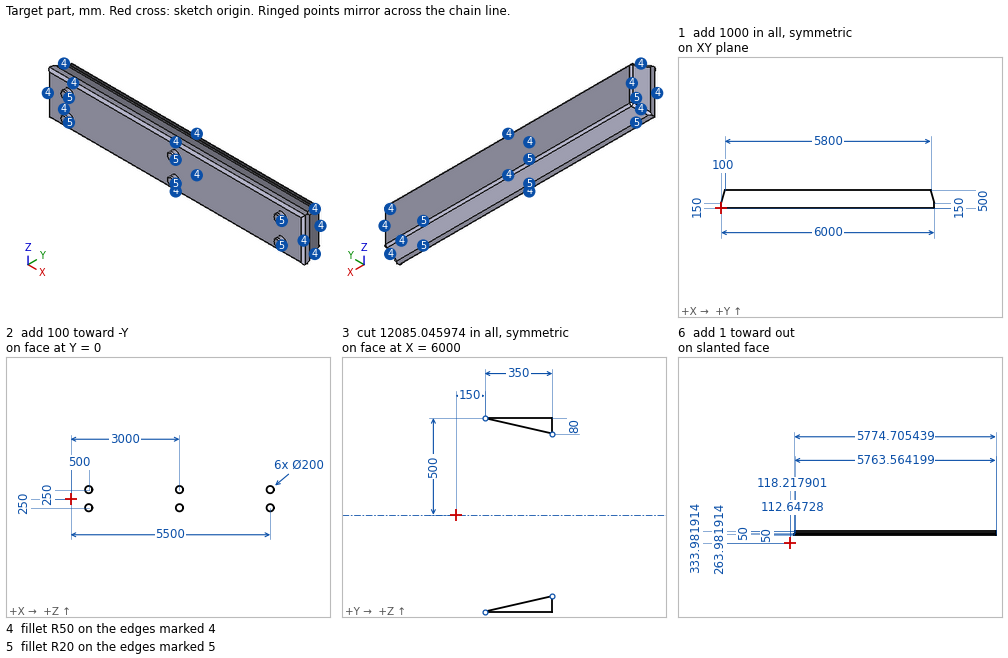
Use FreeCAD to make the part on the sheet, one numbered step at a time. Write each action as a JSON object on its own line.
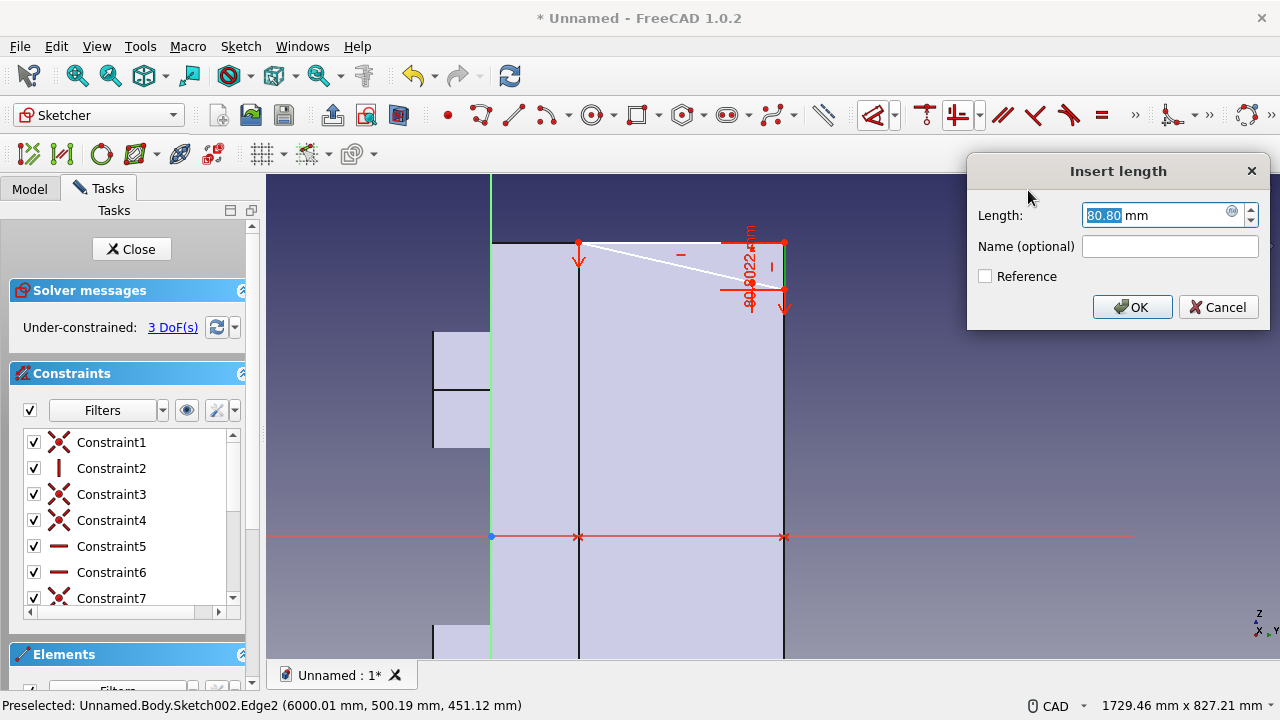
{"action": "type", "text": "80"}
{"action": "key", "text": "Return"}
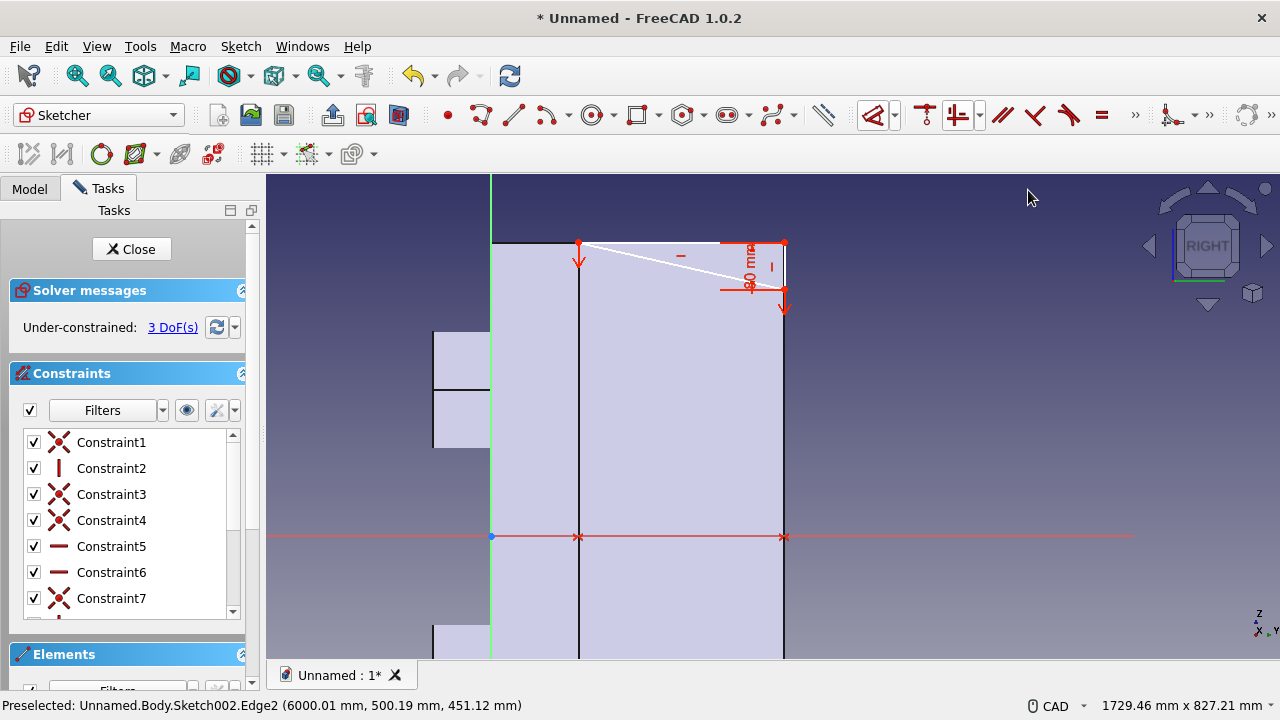
{"action": "left_click", "coordinate": [723, 243]}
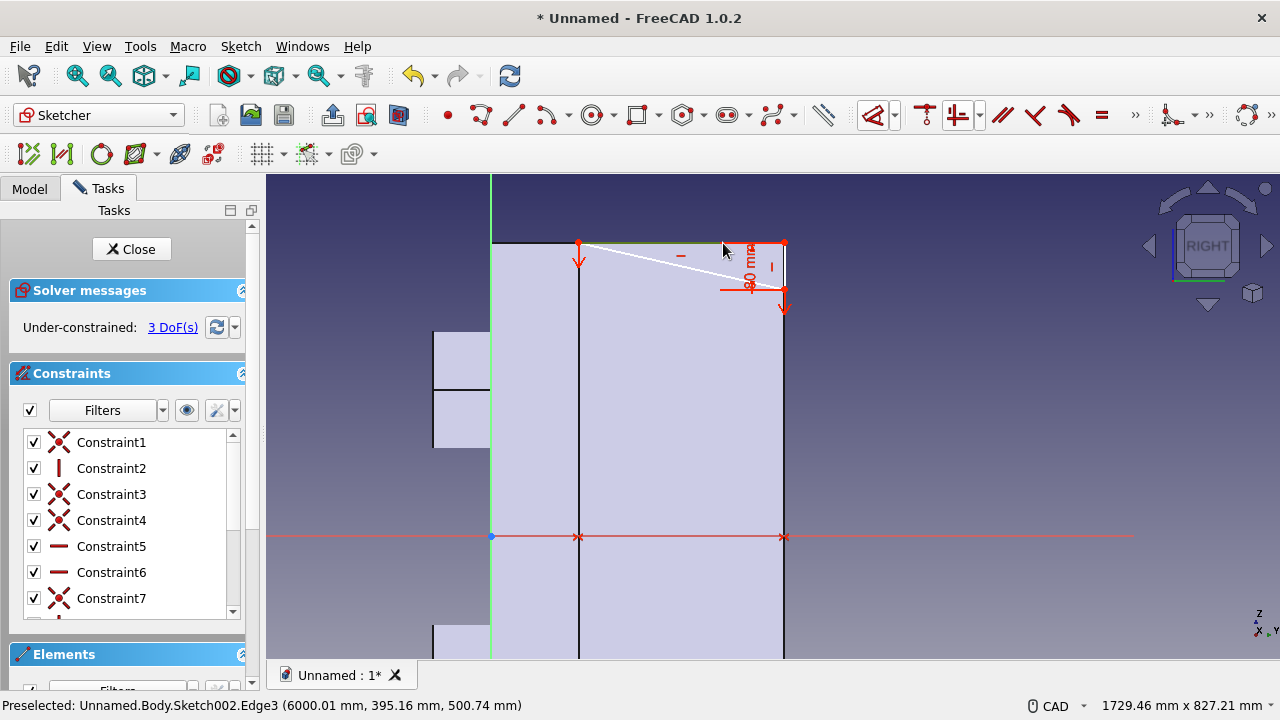
{"action": "key", "text": "l"}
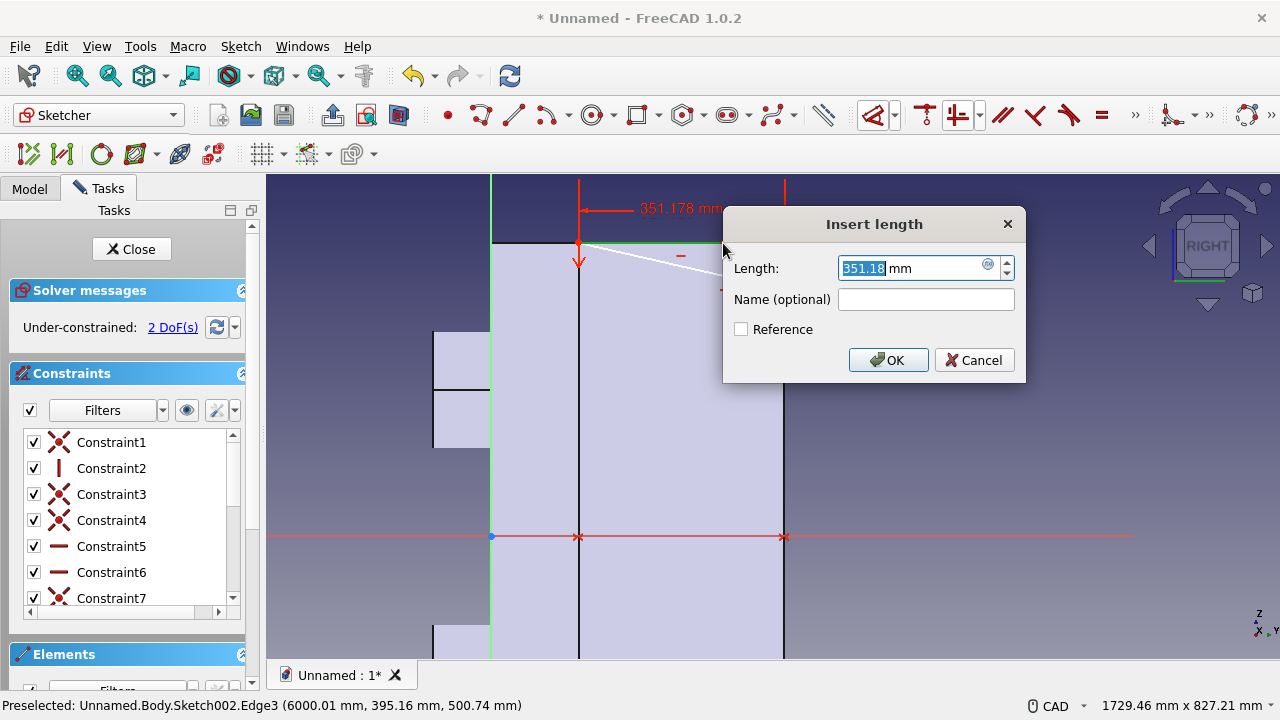
{"action": "type", "text": "350"}
{"action": "key", "text": "Return"}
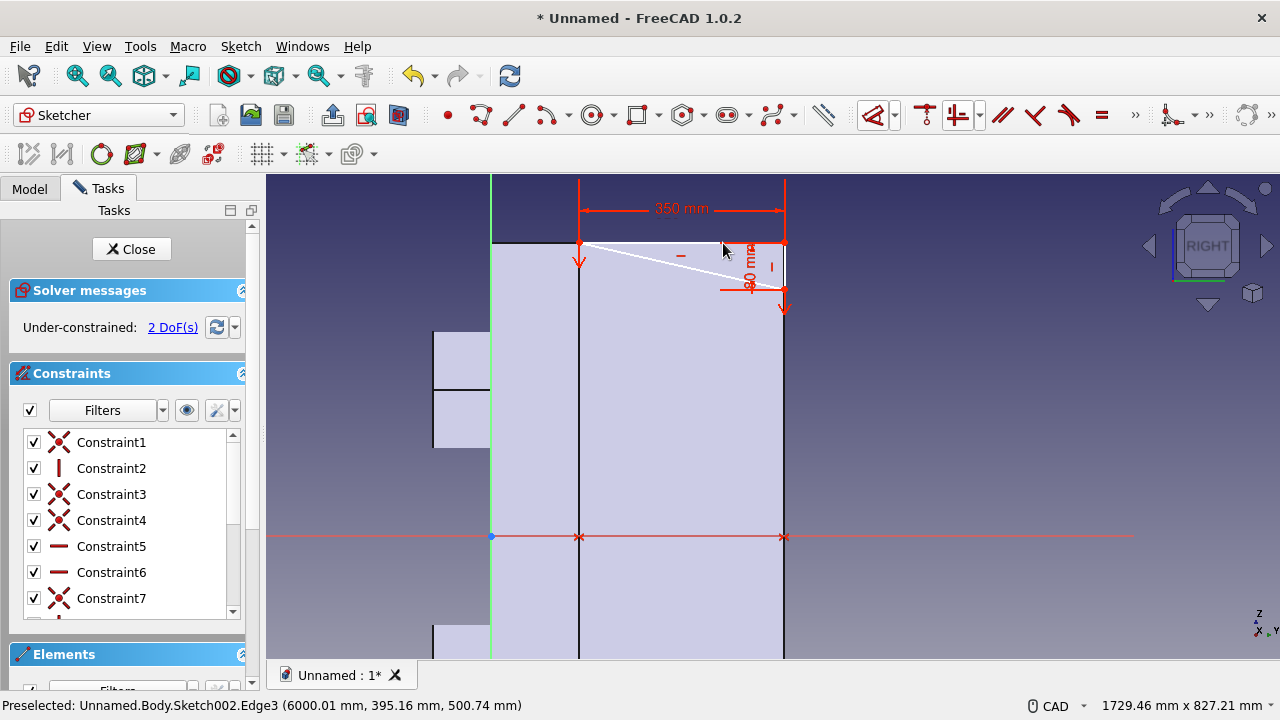
{"action": "left_click", "coordinate": [579, 243]}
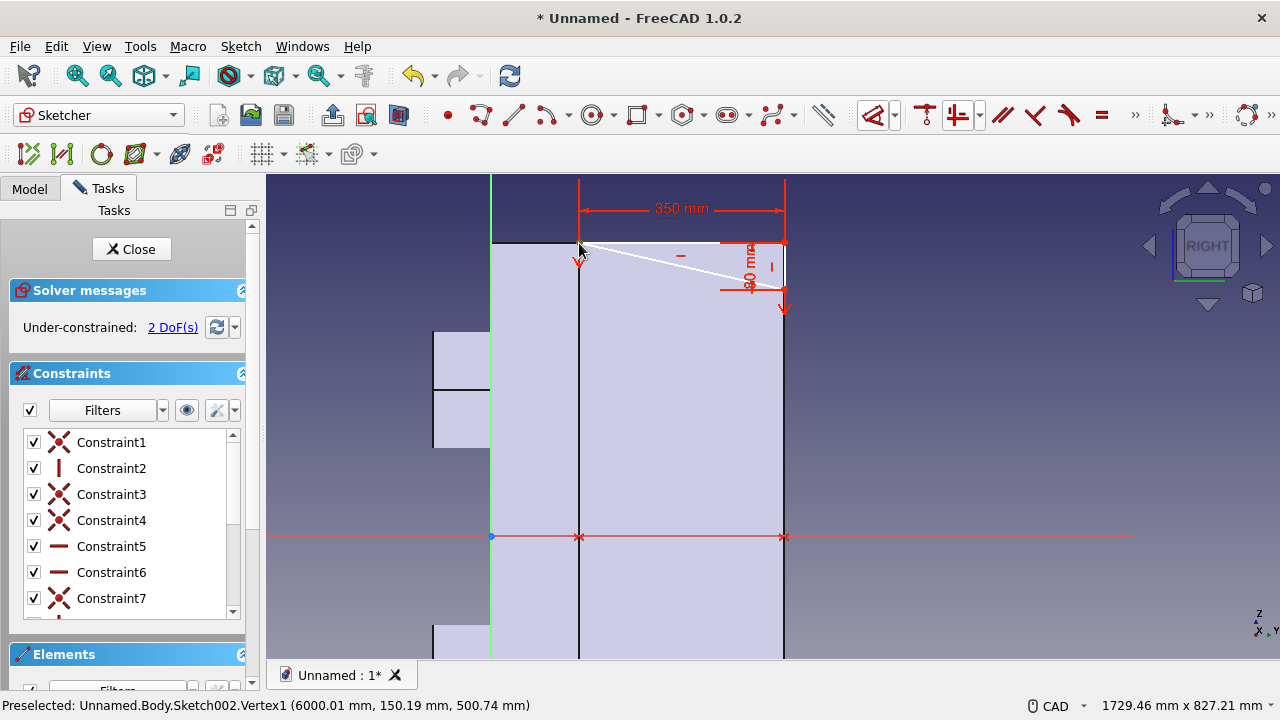
{"action": "left_click", "coordinate": [894, 116]}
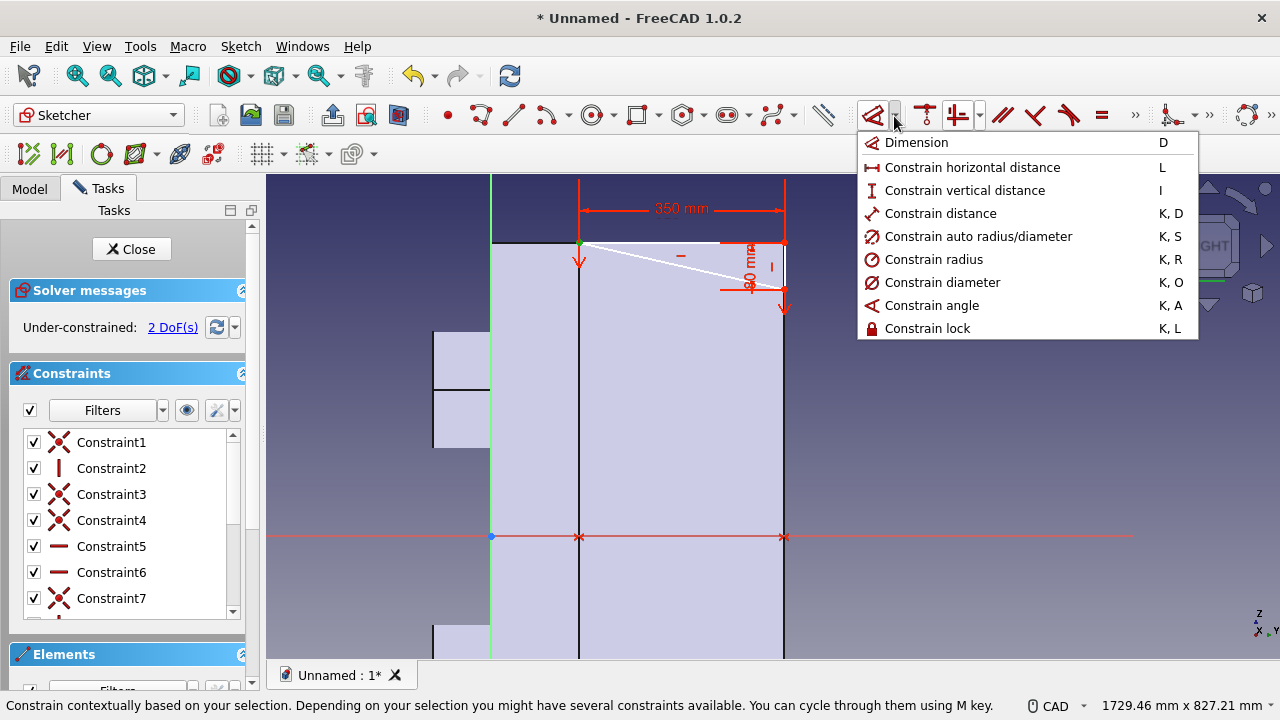
{"action": "left_click", "coordinate": [1028, 168]}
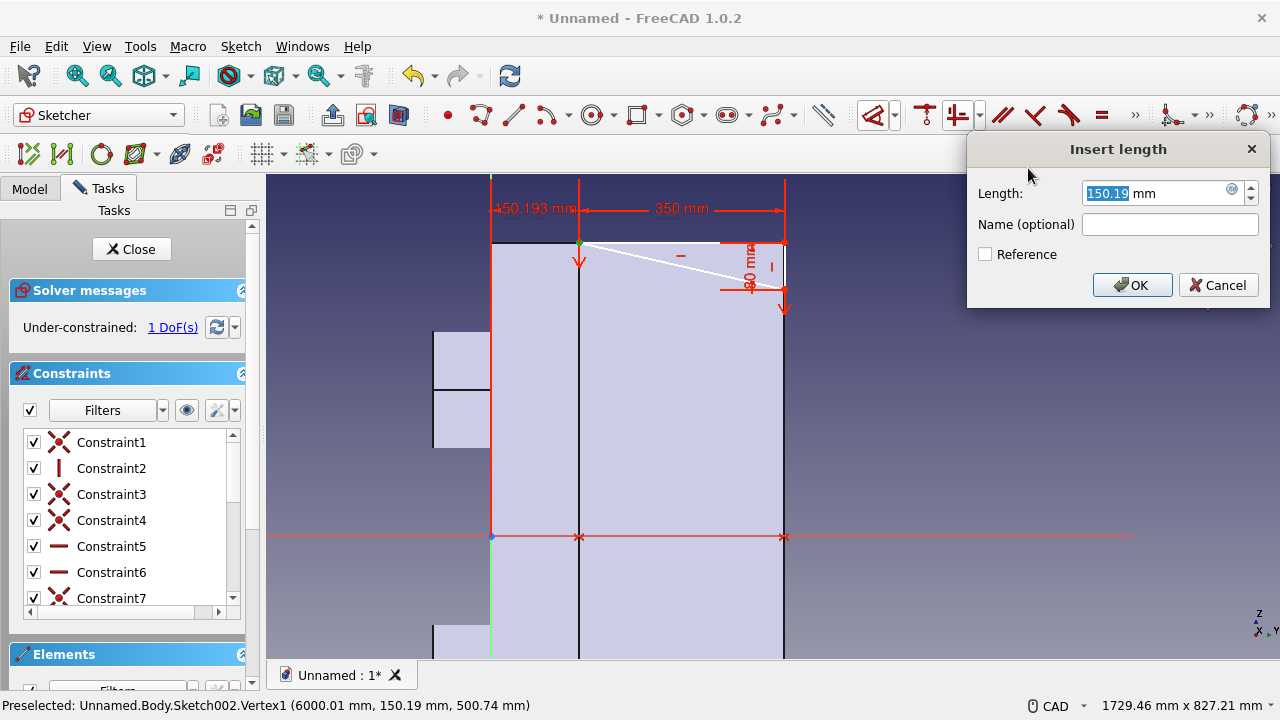
{"action": "type", "text": "150"}
{"action": "key", "text": "Return"}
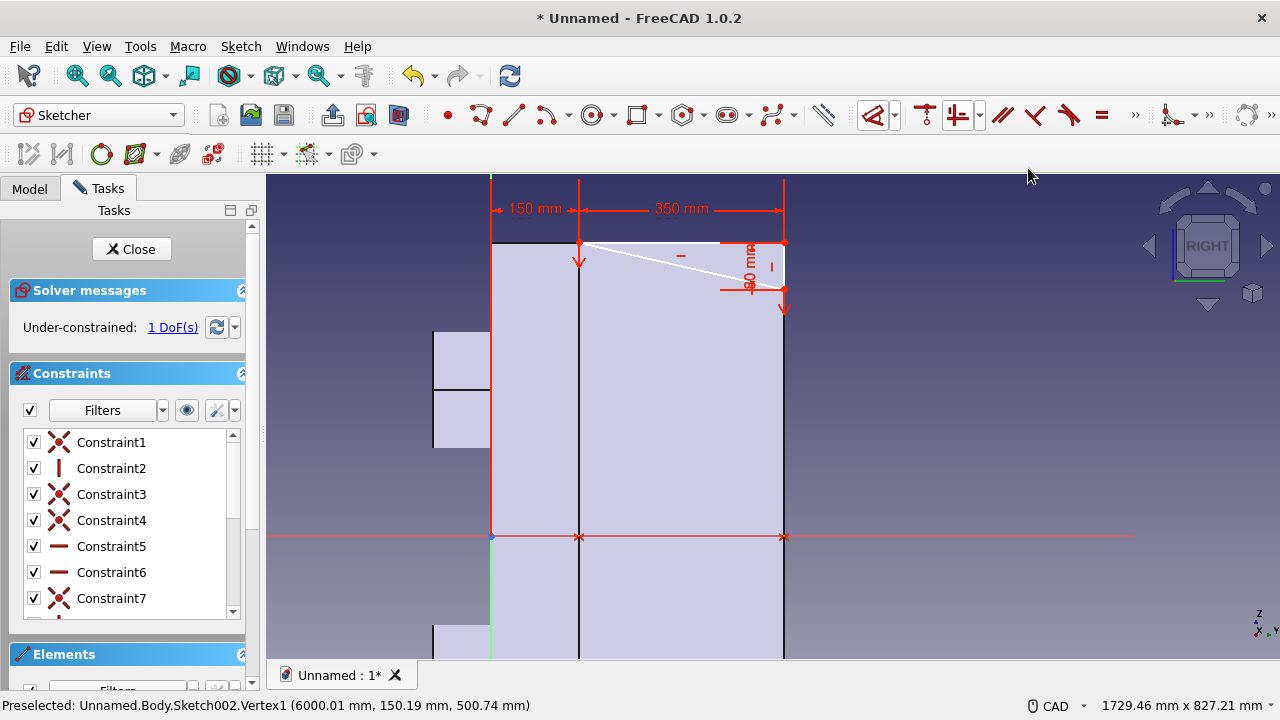
{"action": "left_click", "coordinate": [579, 243]}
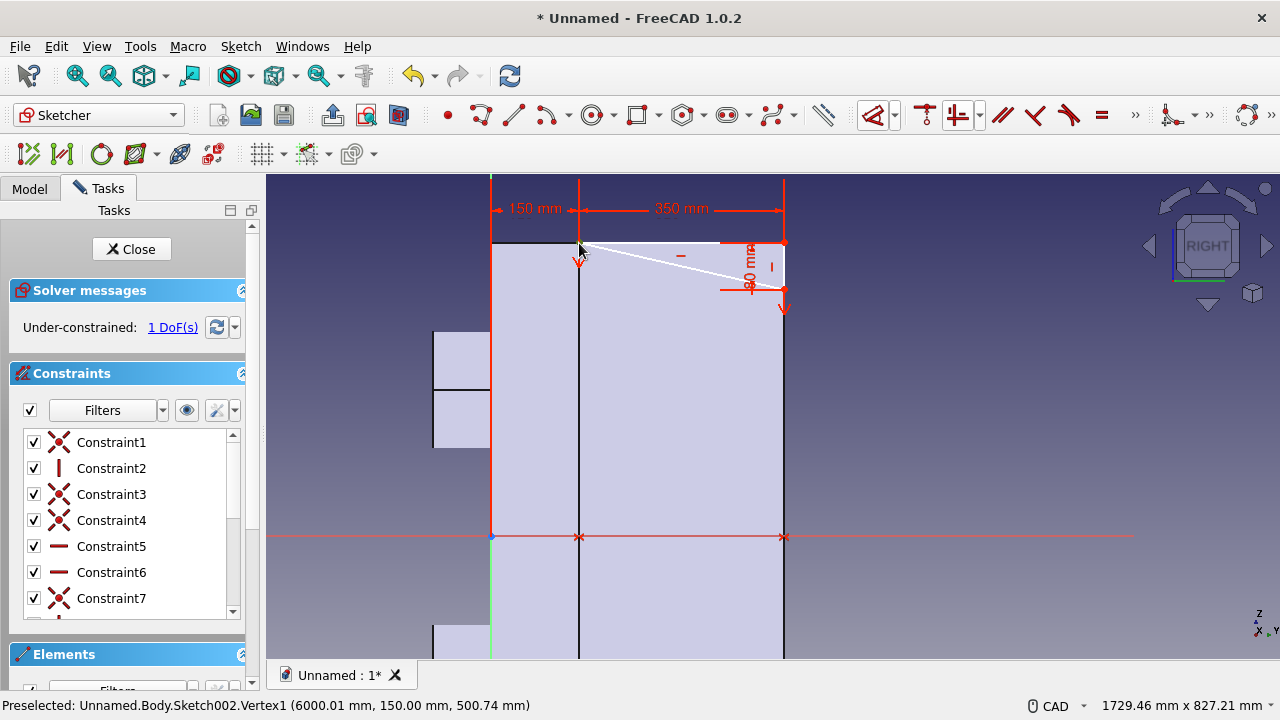
{"action": "key", "text": "i"}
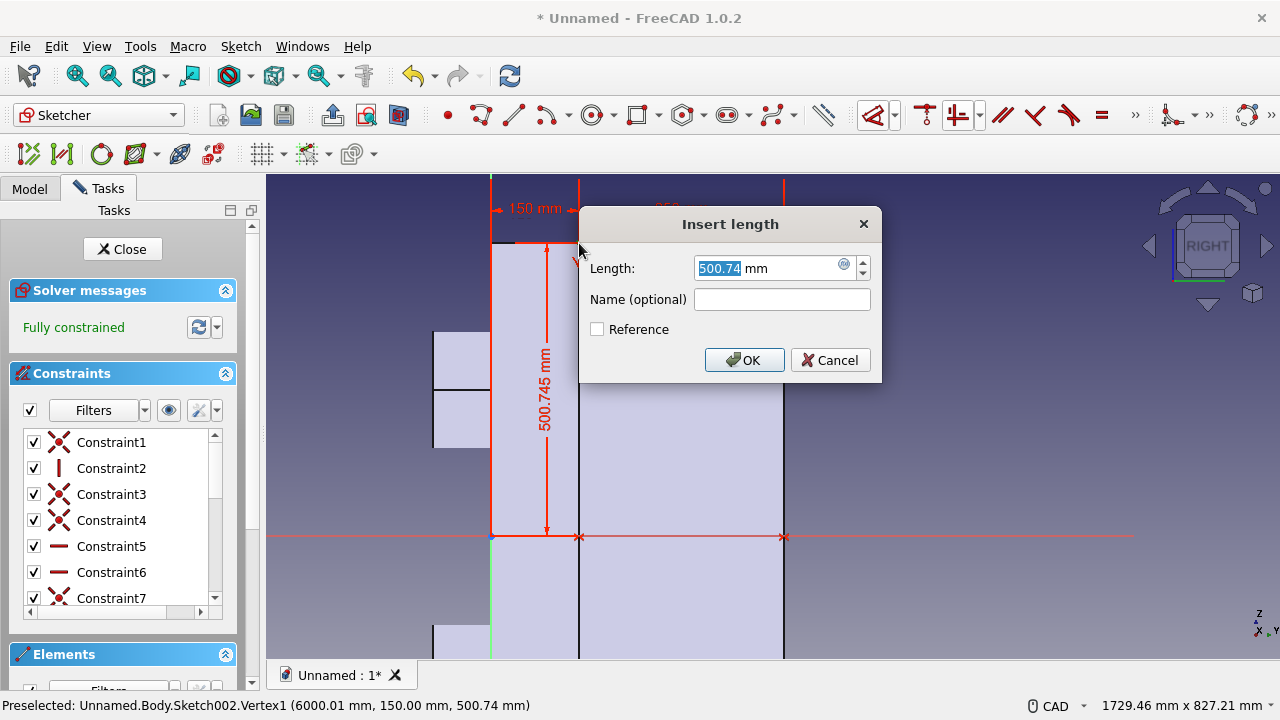
{"action": "type", "text": "500"}
{"action": "key", "text": "Return"}